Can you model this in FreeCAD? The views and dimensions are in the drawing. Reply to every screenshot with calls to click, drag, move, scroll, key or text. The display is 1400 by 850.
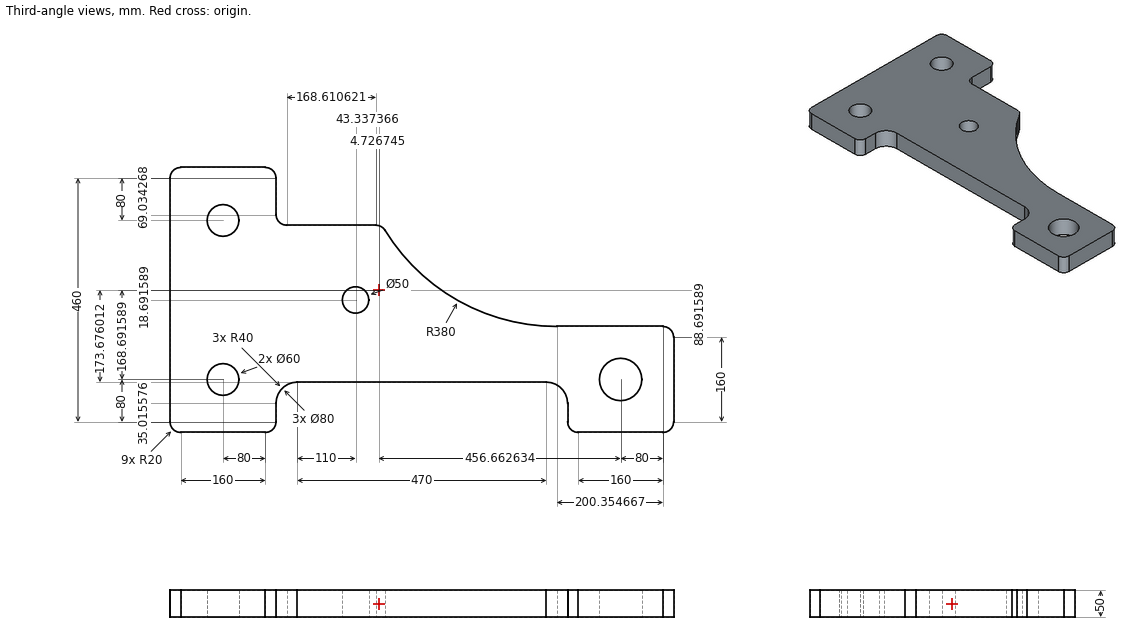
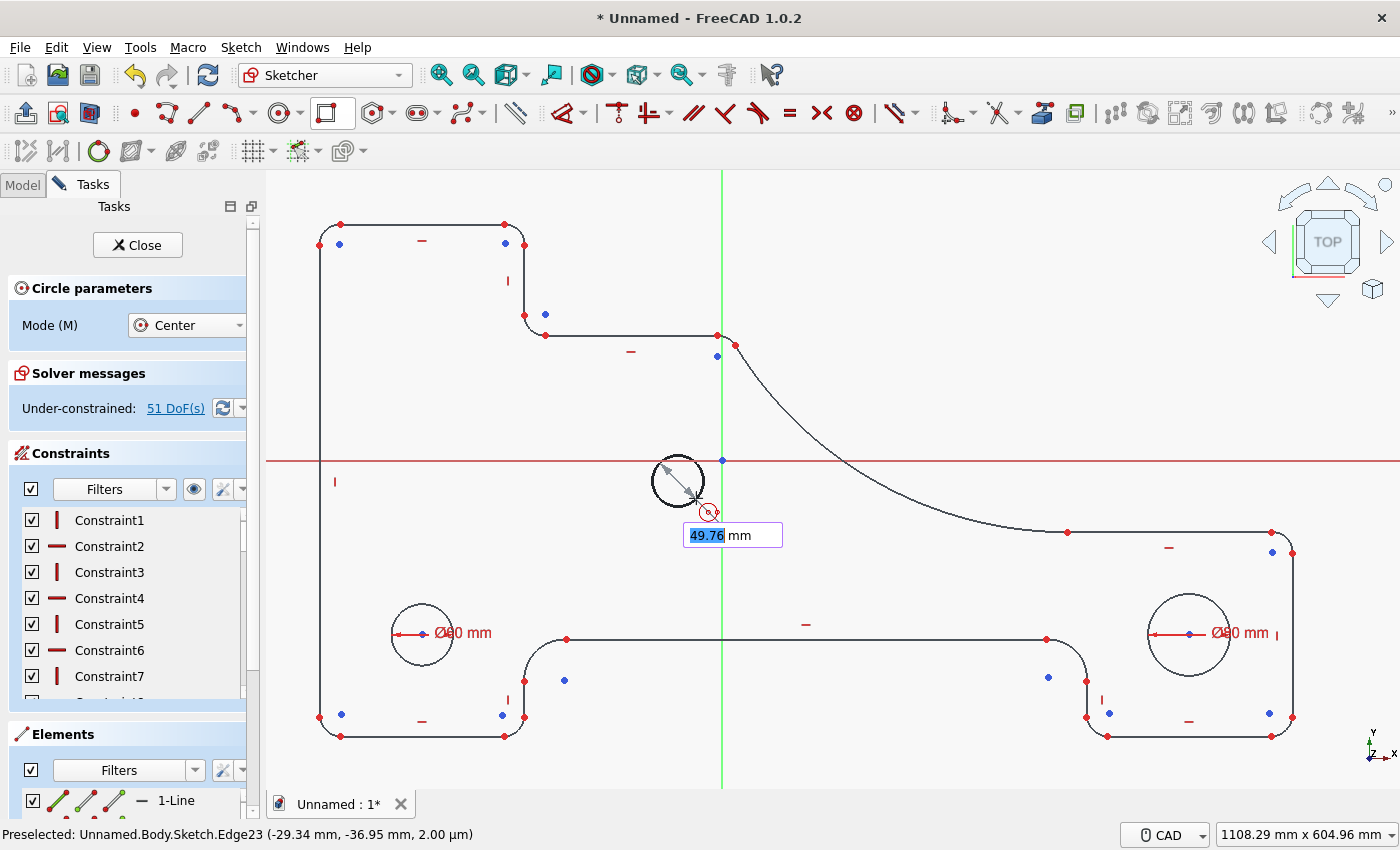
text(50)
key(Return)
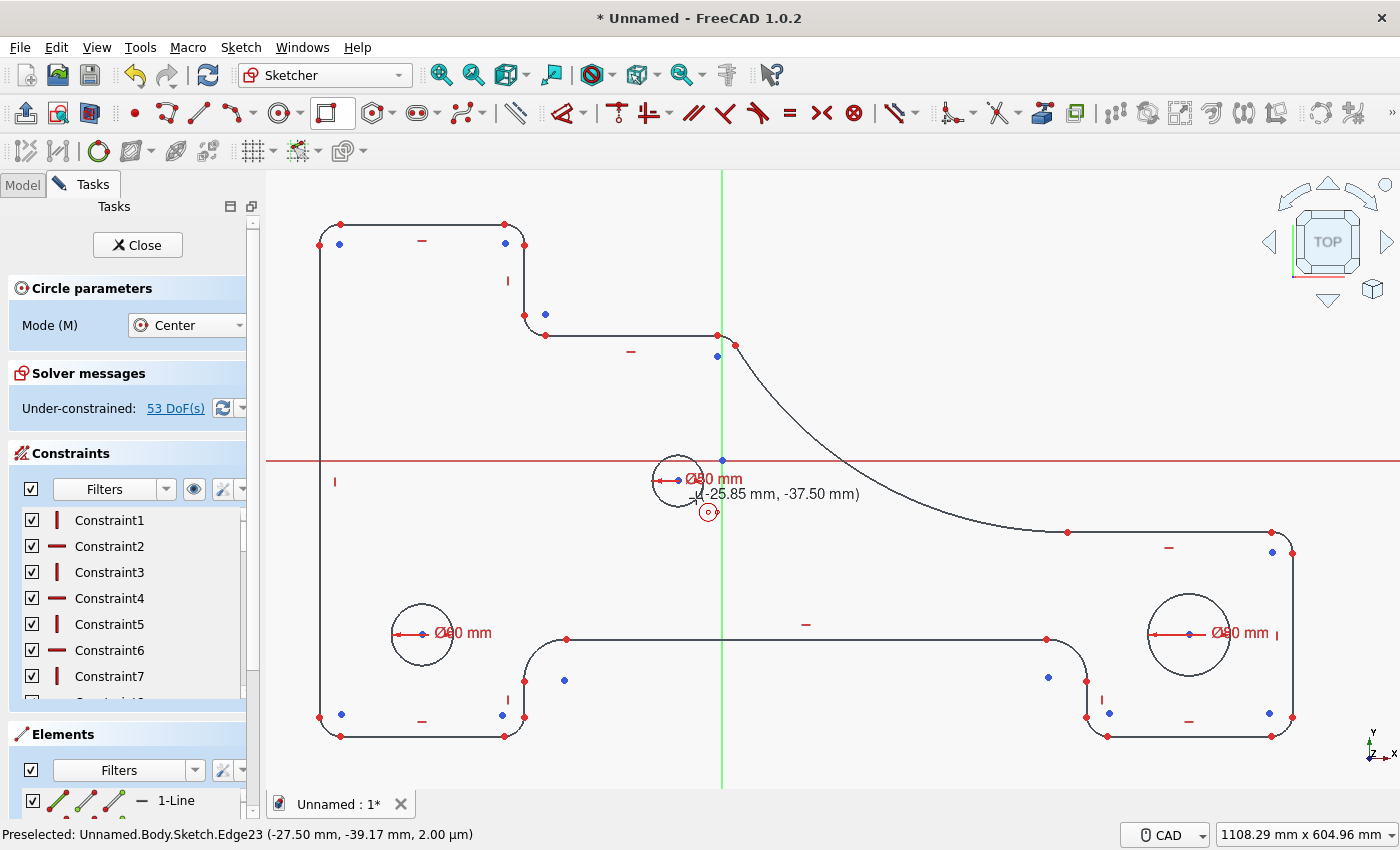
click(422, 326)
move(444, 305)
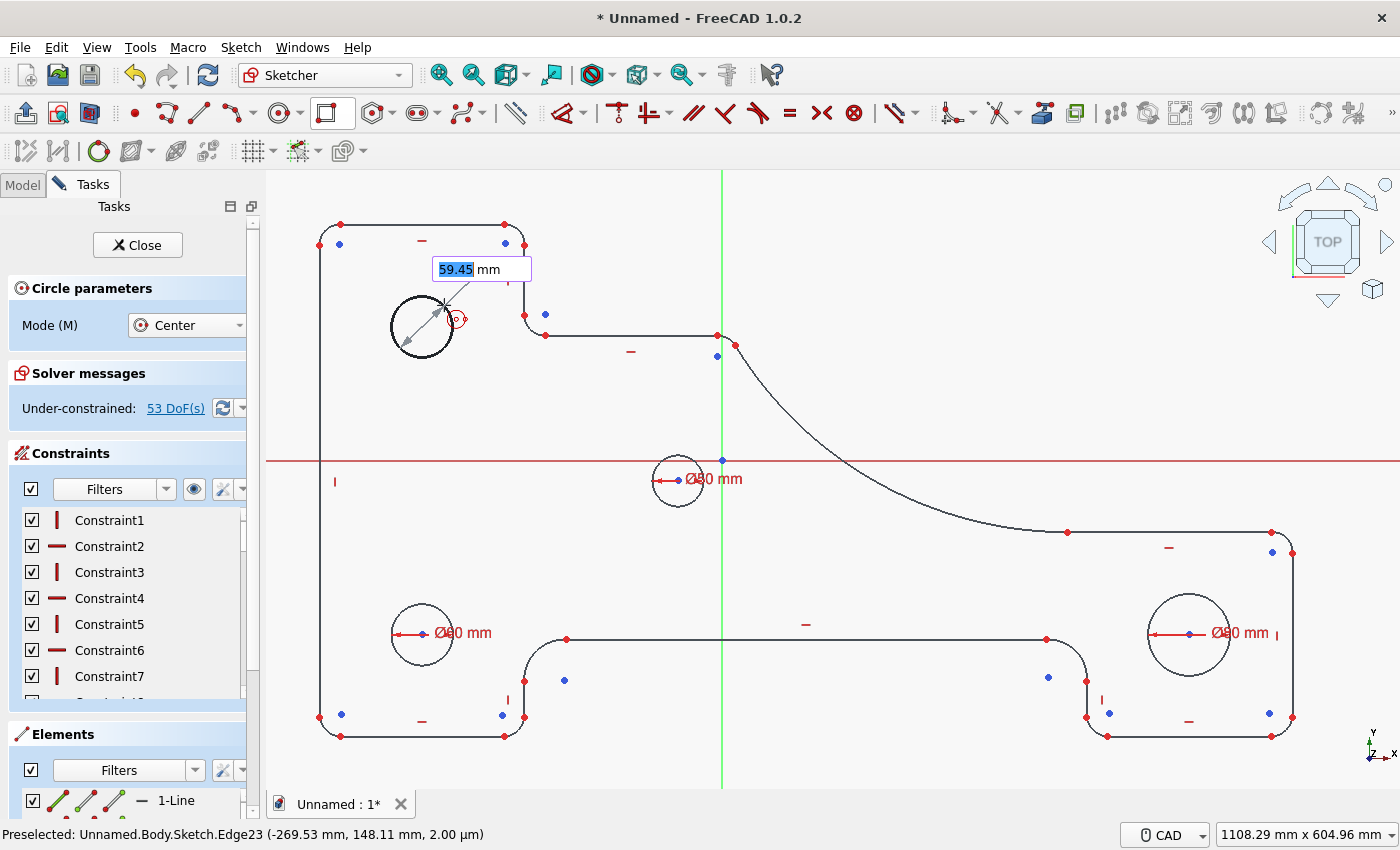
text(60)
key(Return)
key(Escape)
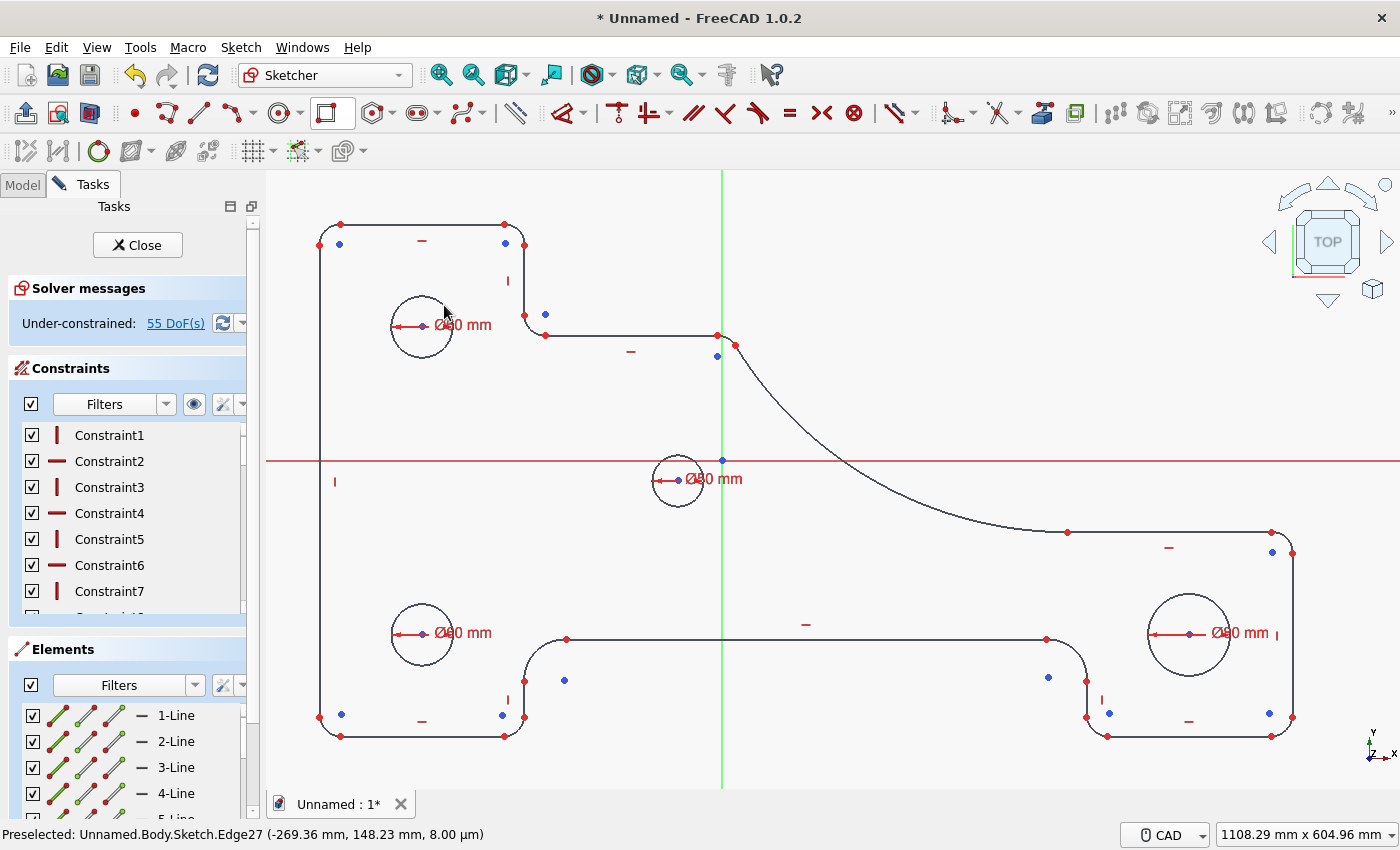
click(320, 387)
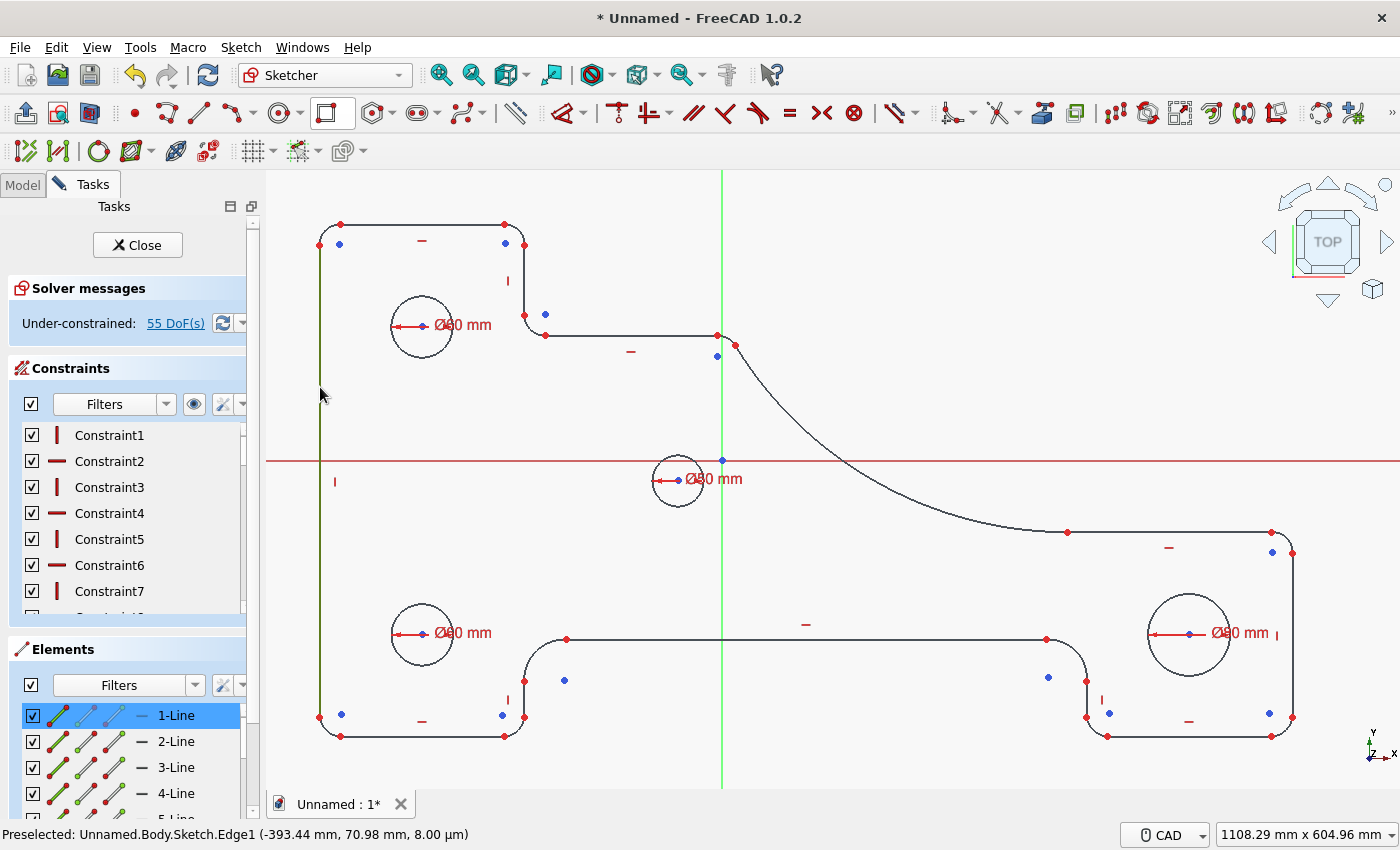
scroll(323, 726, up, 3)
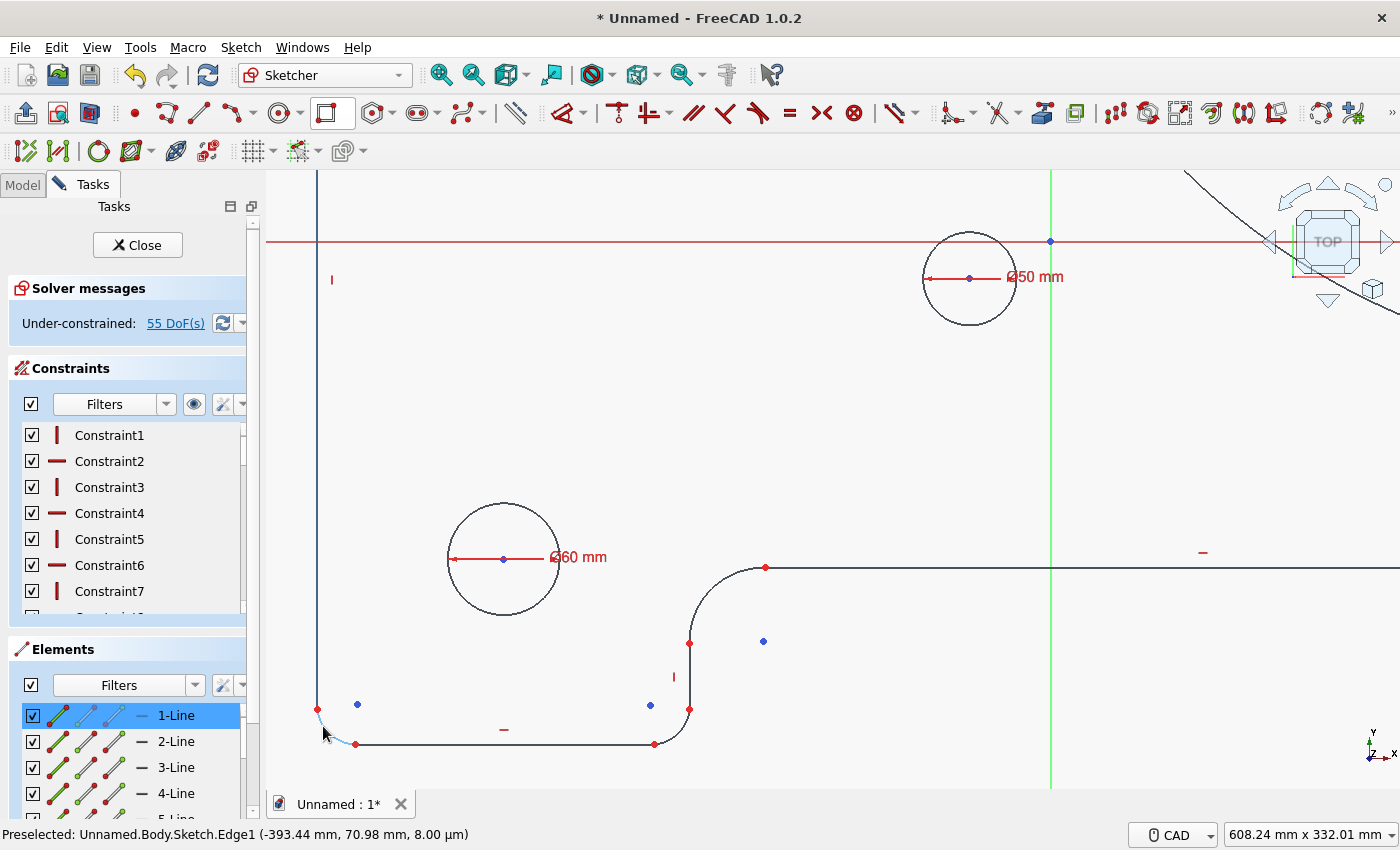
click(323, 725)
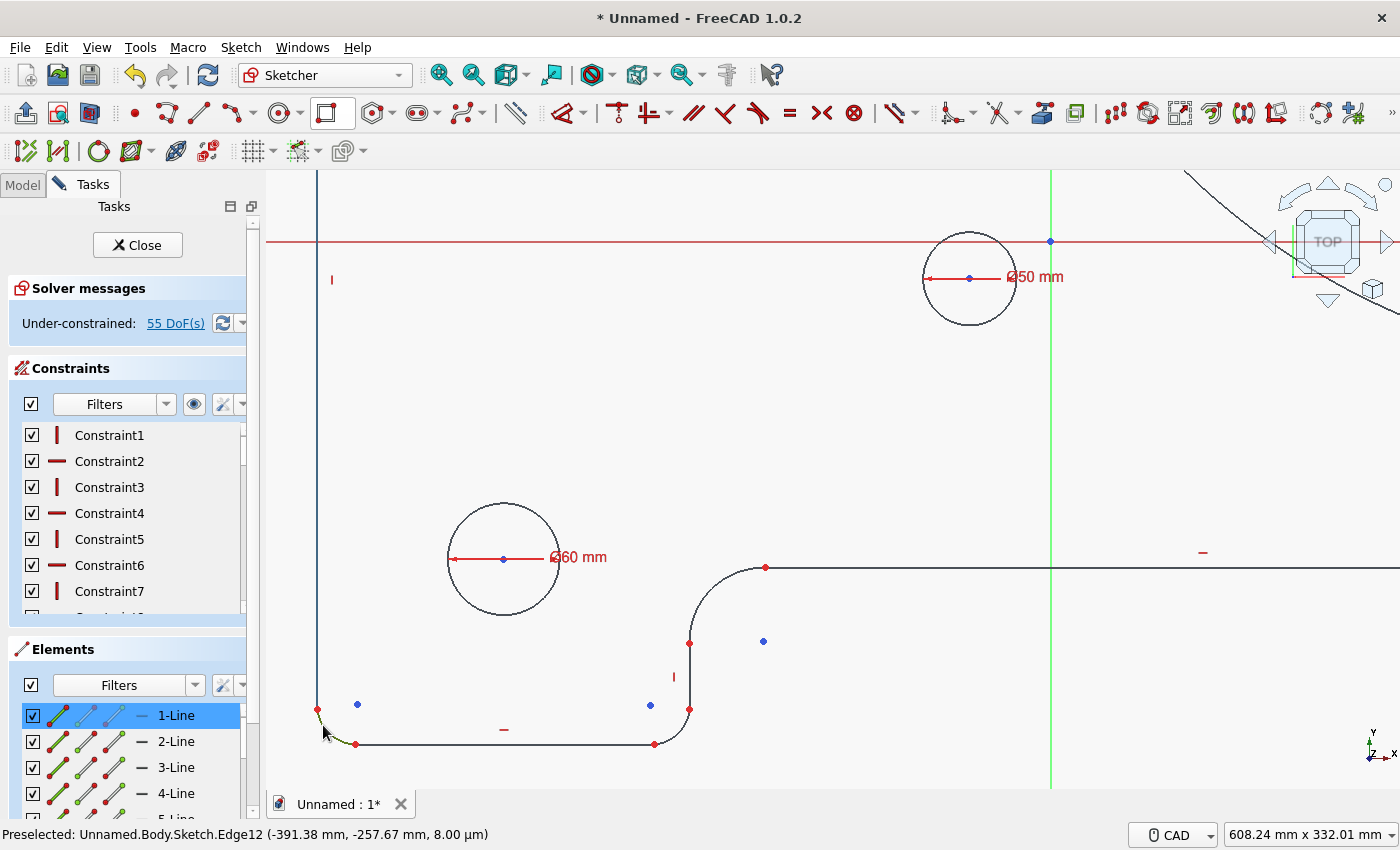
click(758, 114)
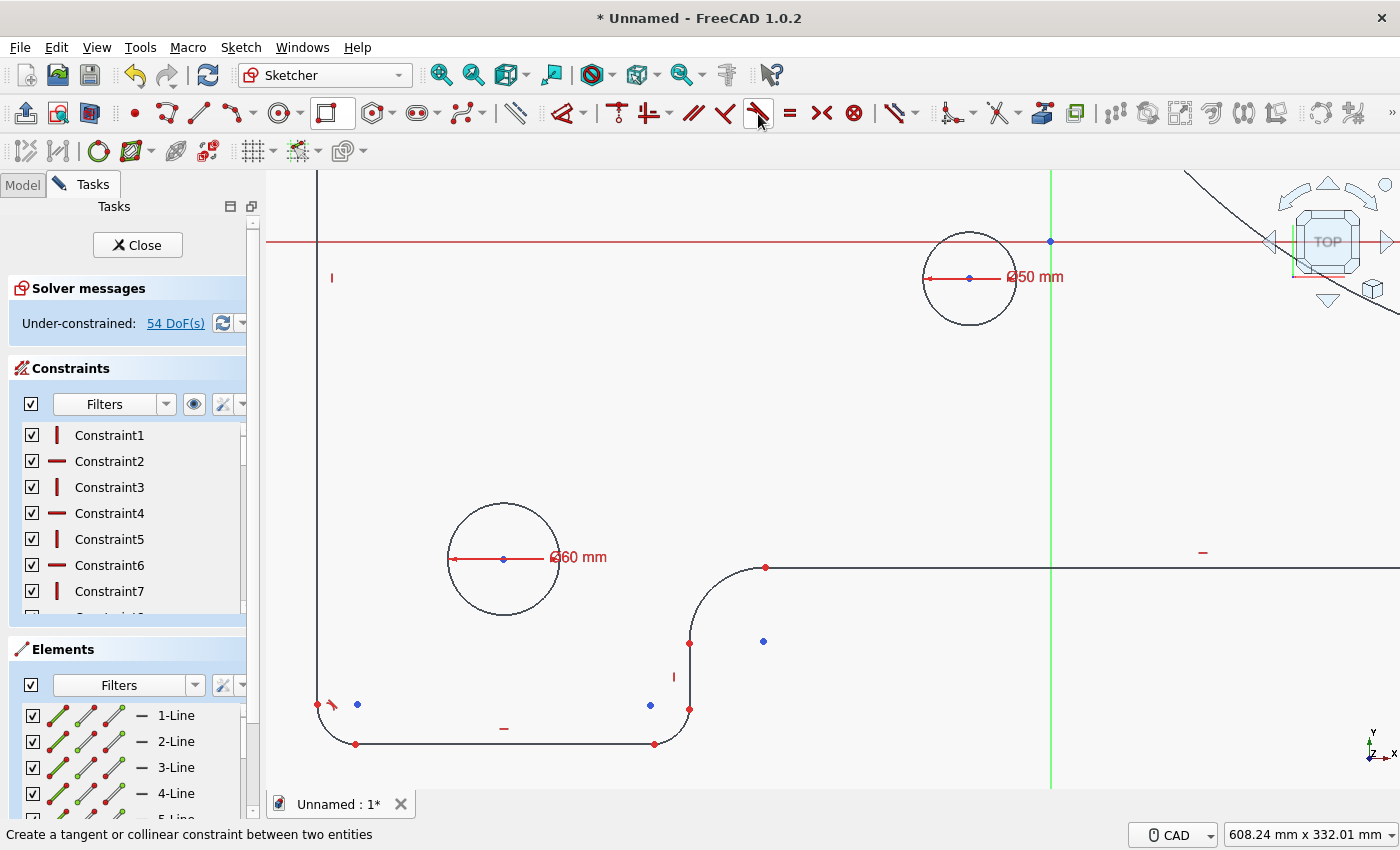
click(317, 448)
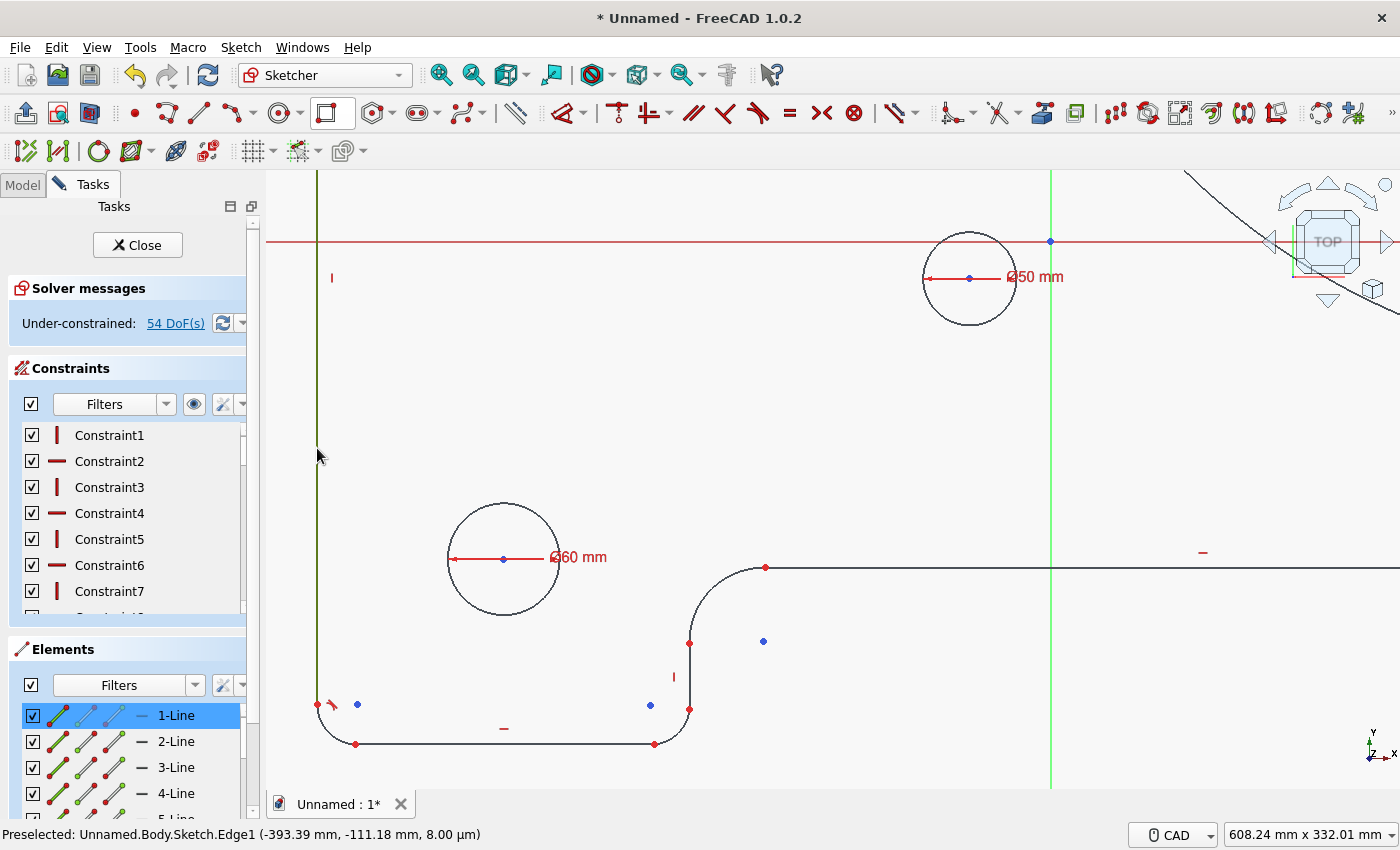
scroll(509, 598, down, 5)